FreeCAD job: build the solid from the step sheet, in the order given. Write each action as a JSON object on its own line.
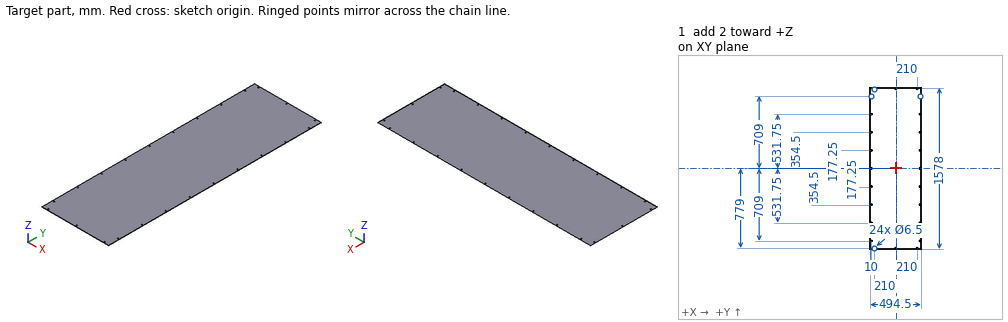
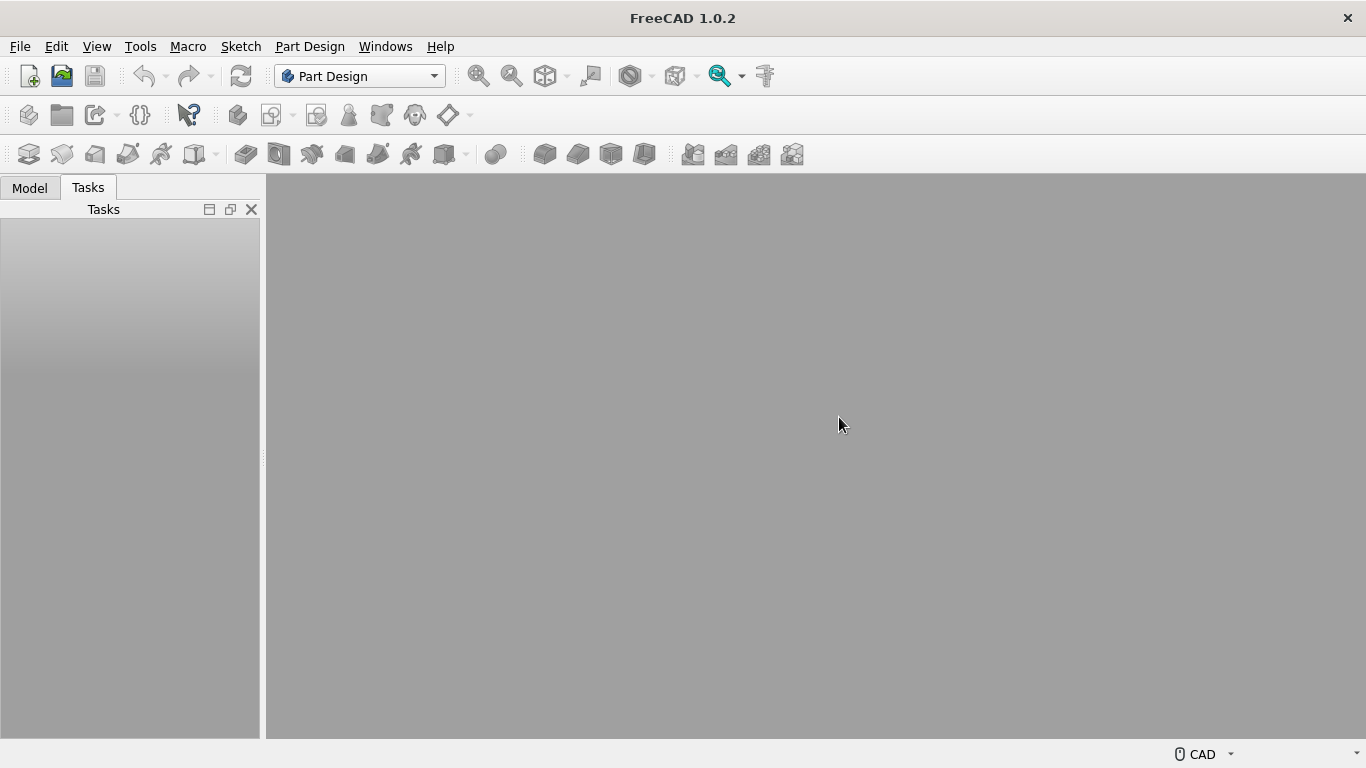
{"action": "key", "text": "ctrl+n"}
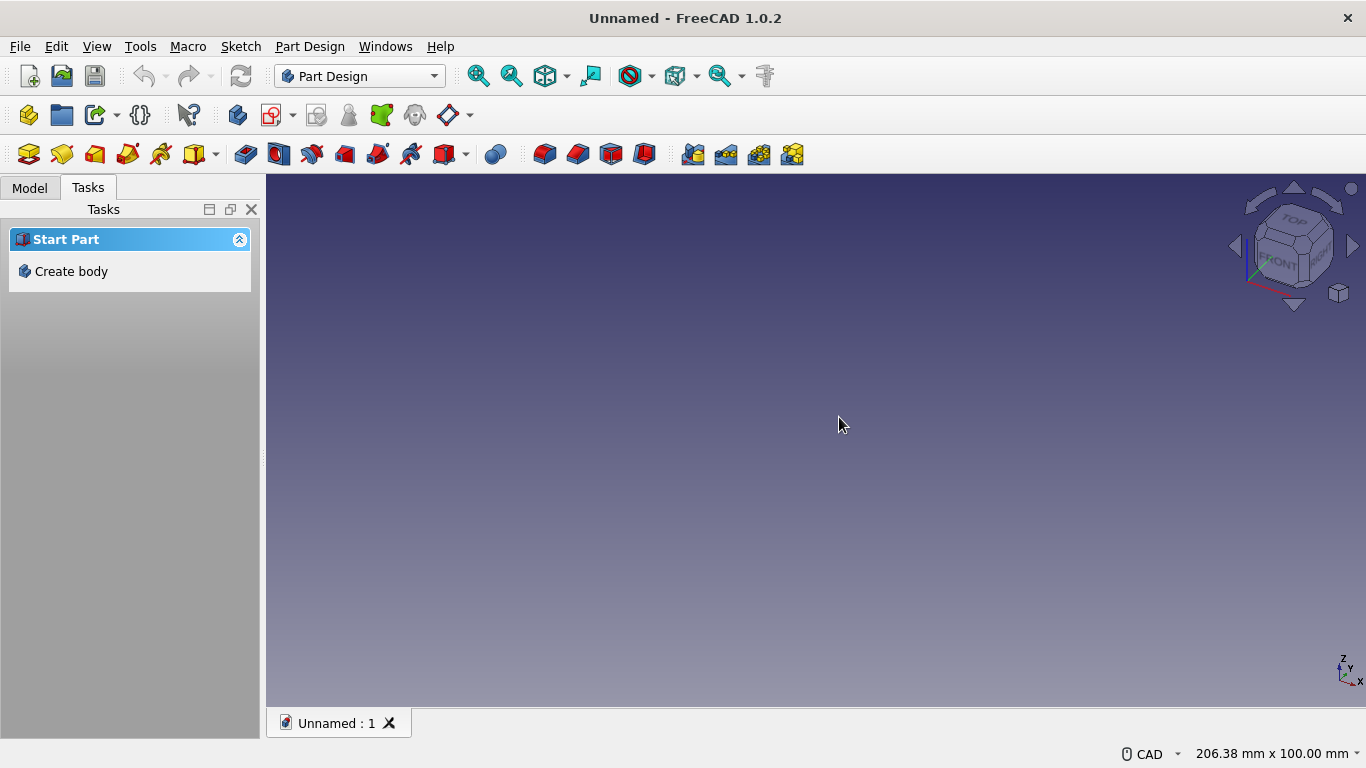
{"action": "left_click", "coordinate": [270, 116]}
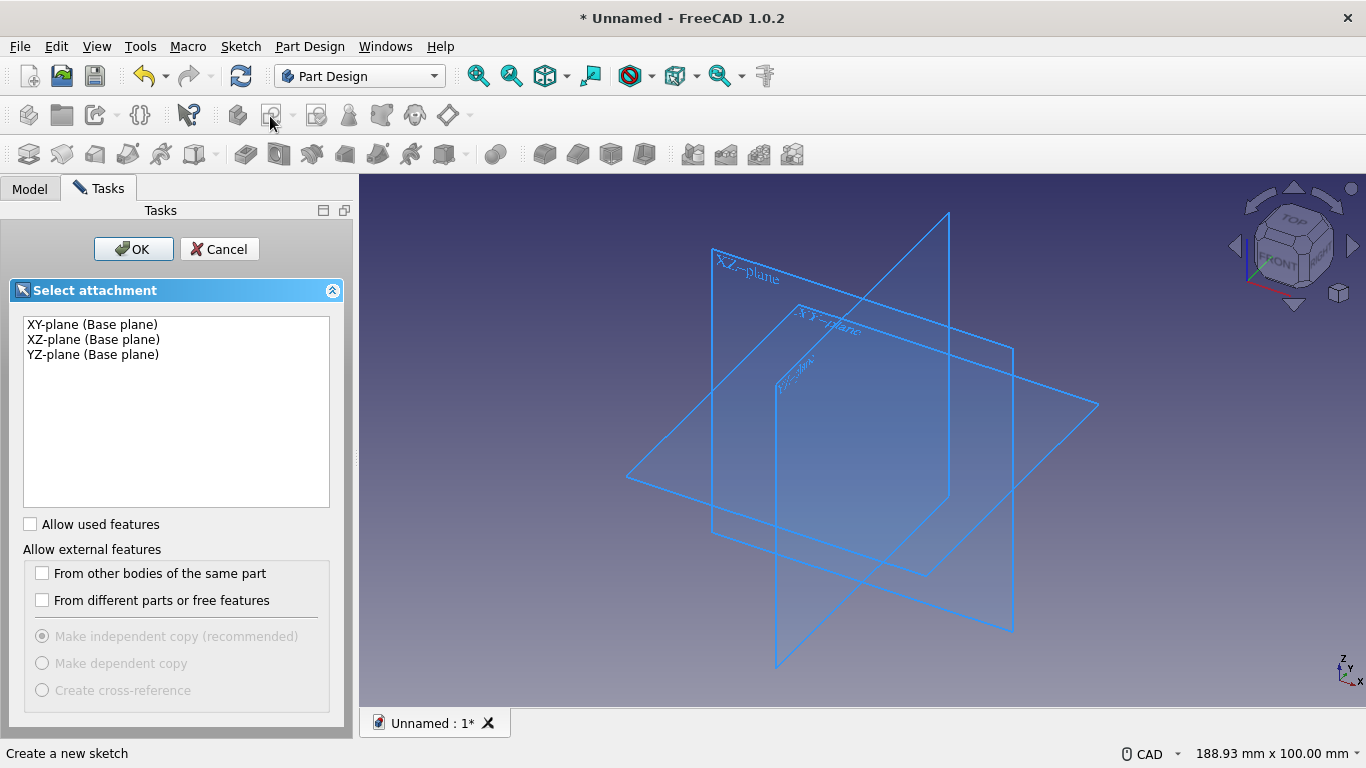
{"action": "left_click", "coordinate": [84, 324]}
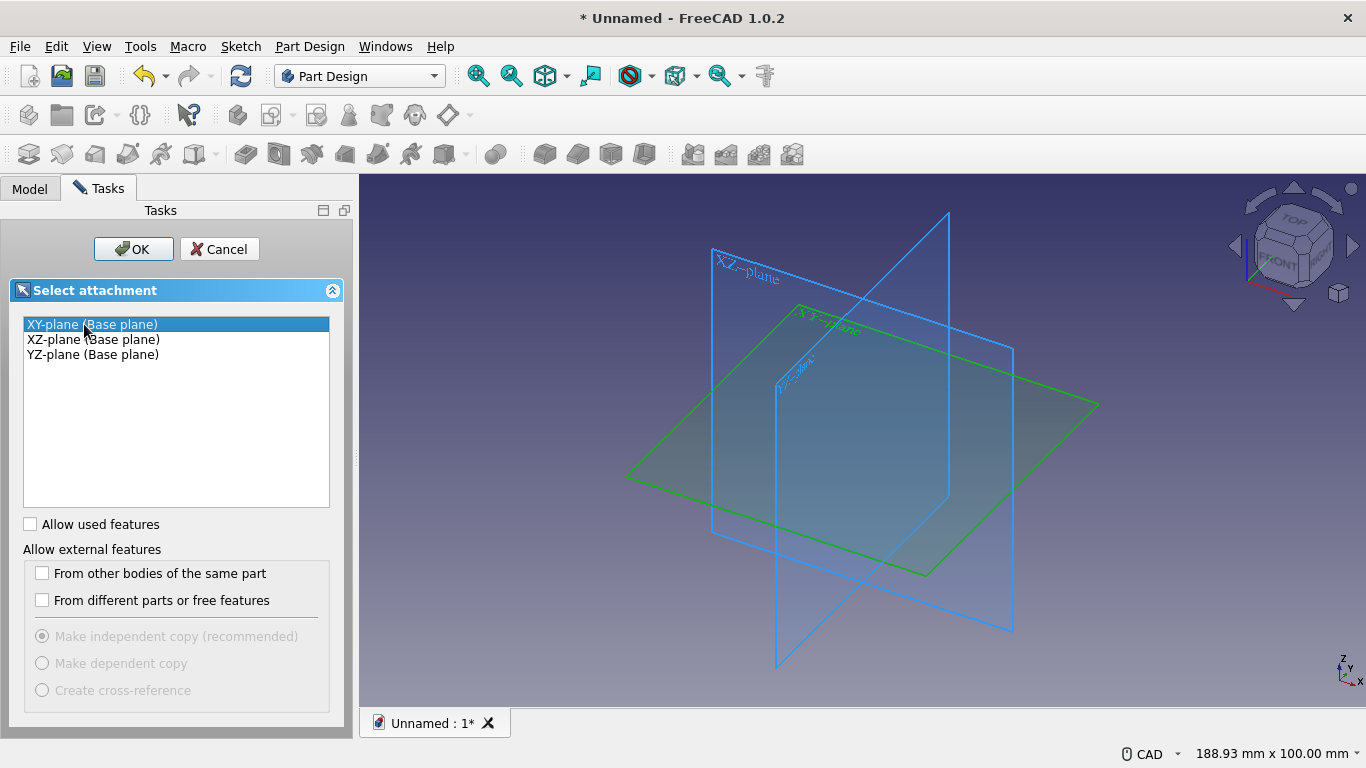
{"action": "left_click", "coordinate": [134, 249]}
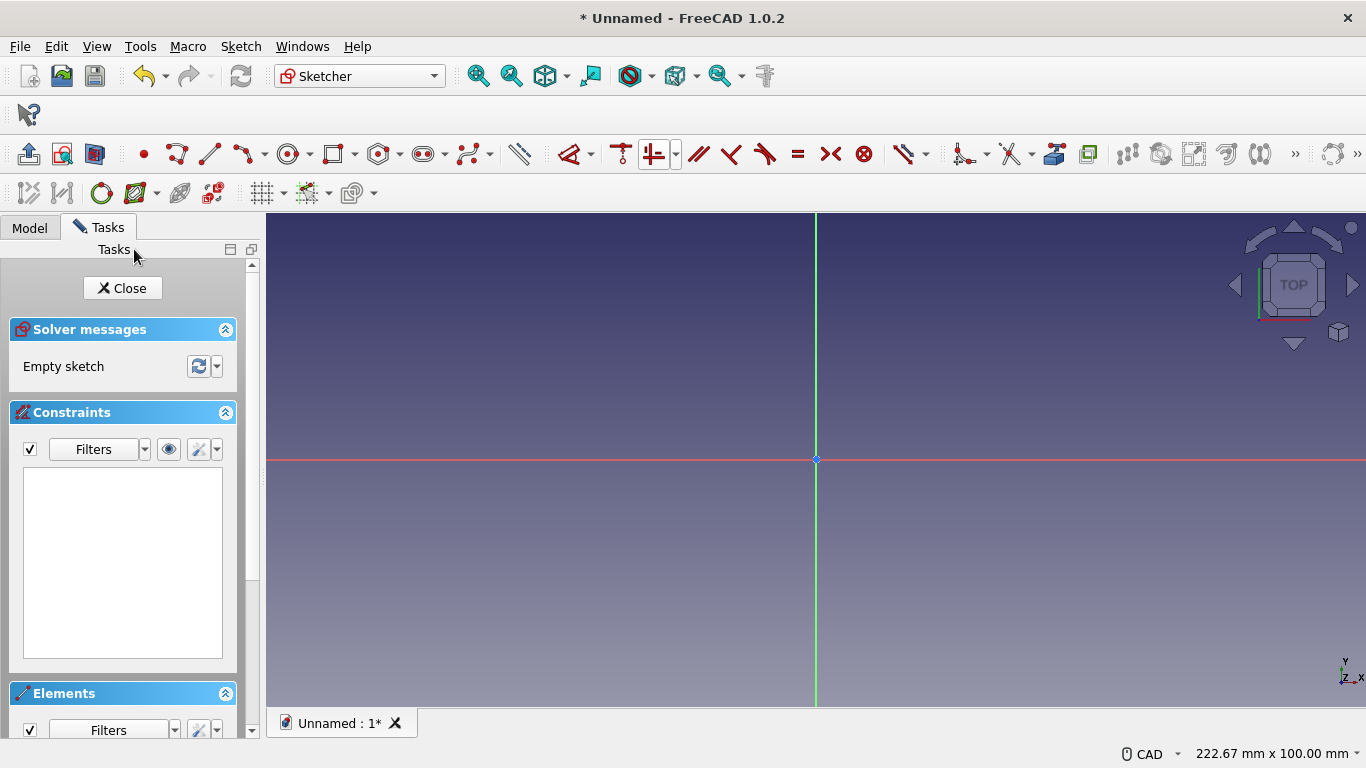
{"action": "scroll", "coordinate": [745, 460], "scroll_direction": "down", "scroll_amount": 16}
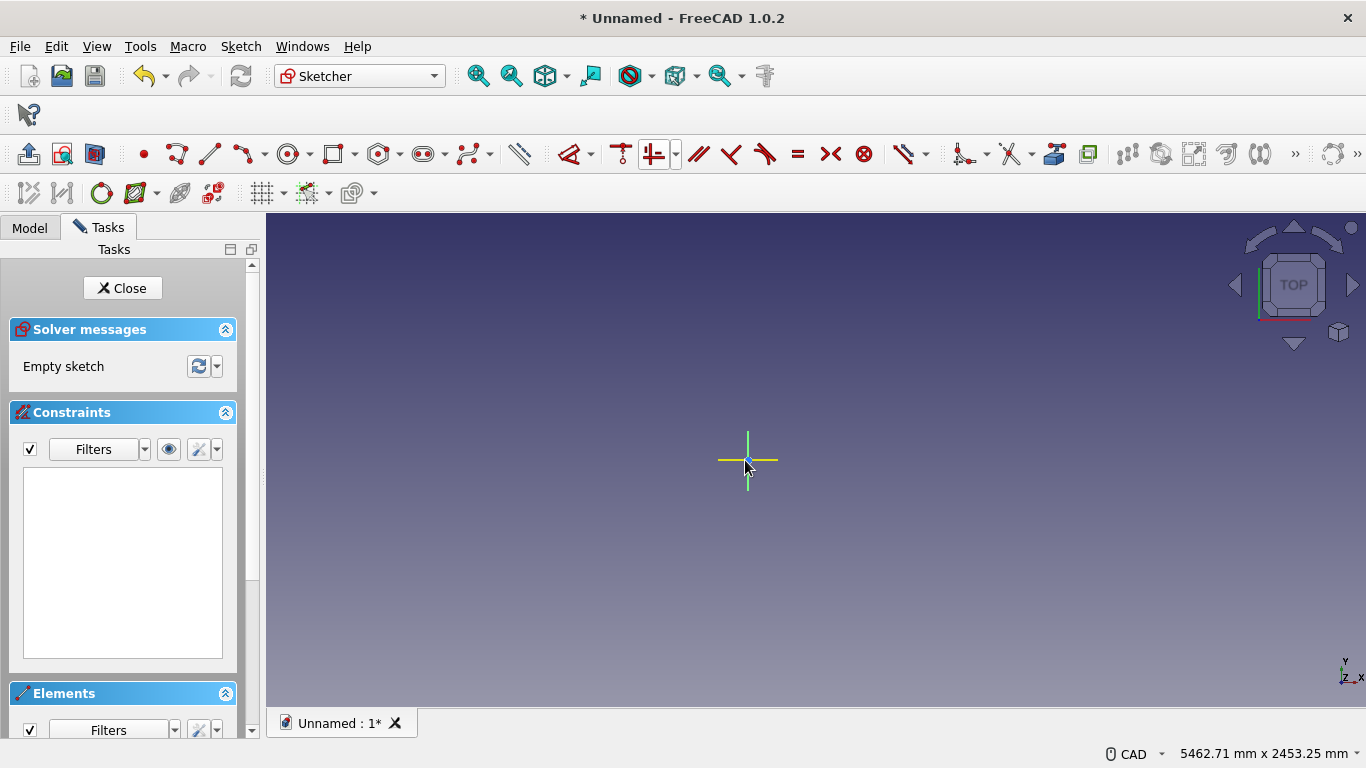
{"action": "key", "text": "g v"}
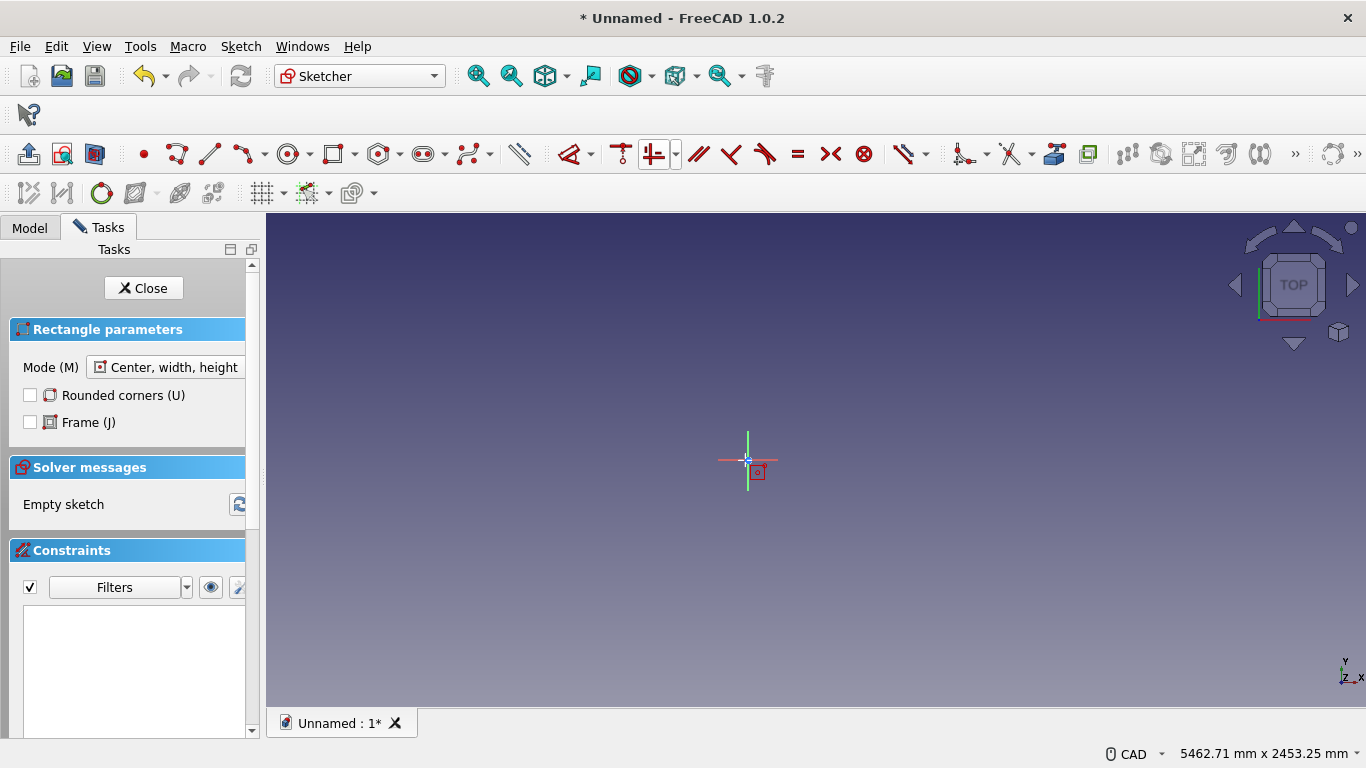
{"action": "left_click", "coordinate": [748, 460]}
{"action": "mouse_move", "coordinate": [798, 302]}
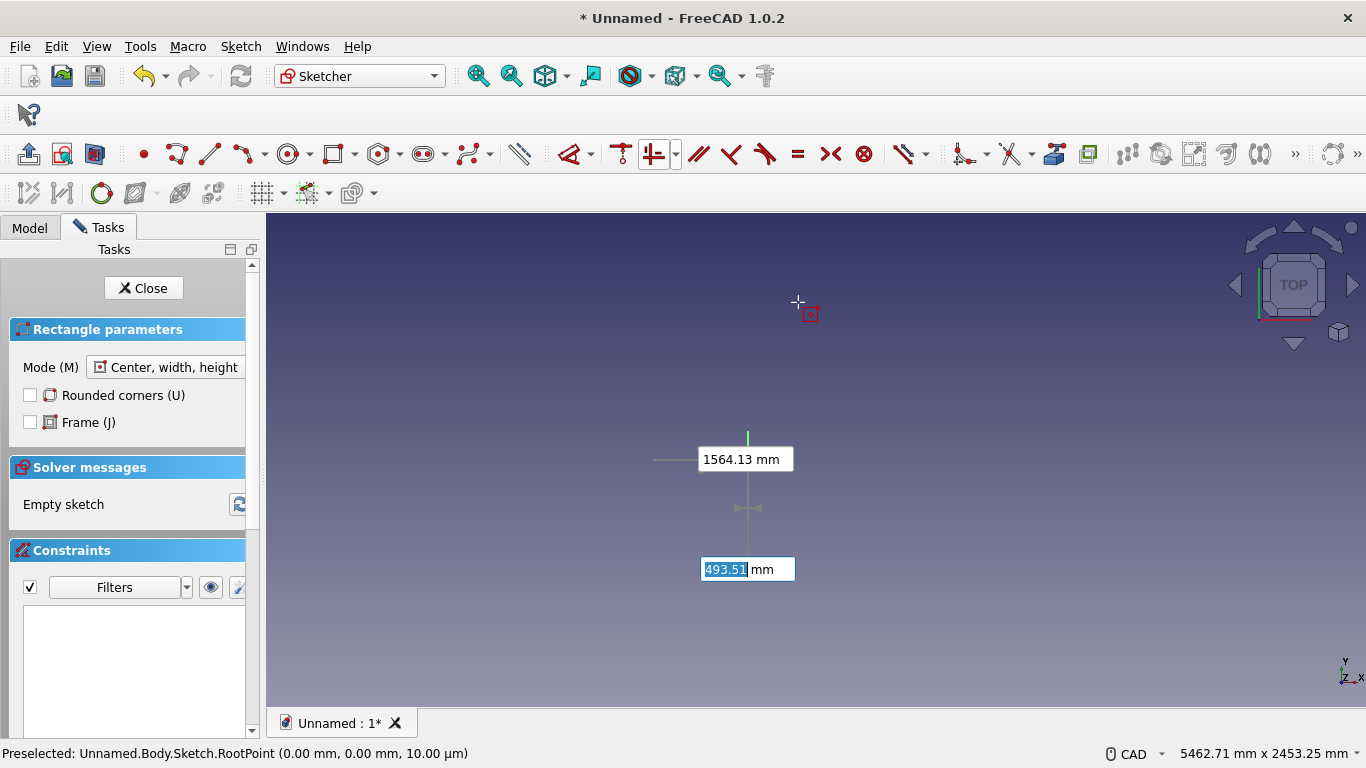
{"action": "type", "text": "494.5"}
{"action": "key", "text": "Tab"}
{"action": "type", "text": "1578"}
{"action": "key", "text": "Return"}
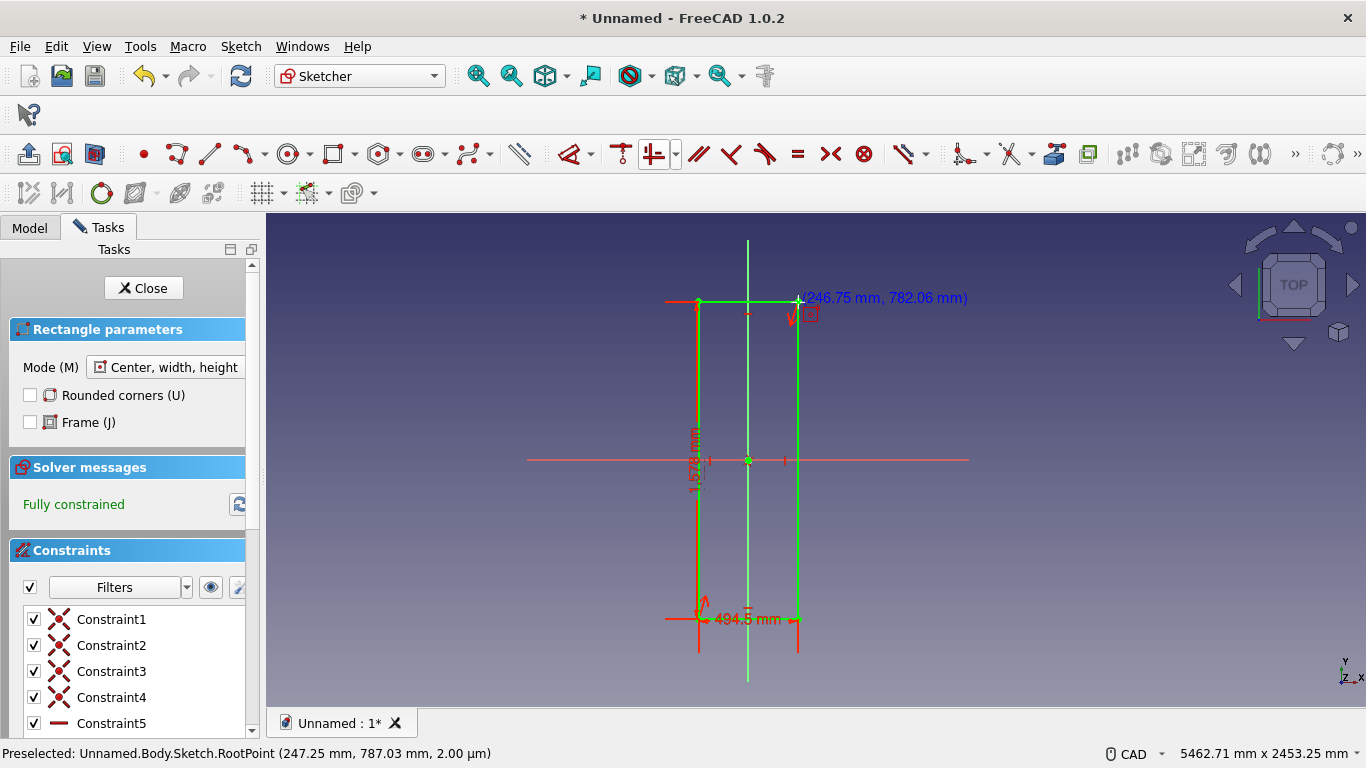
{"action": "key", "text": "g c"}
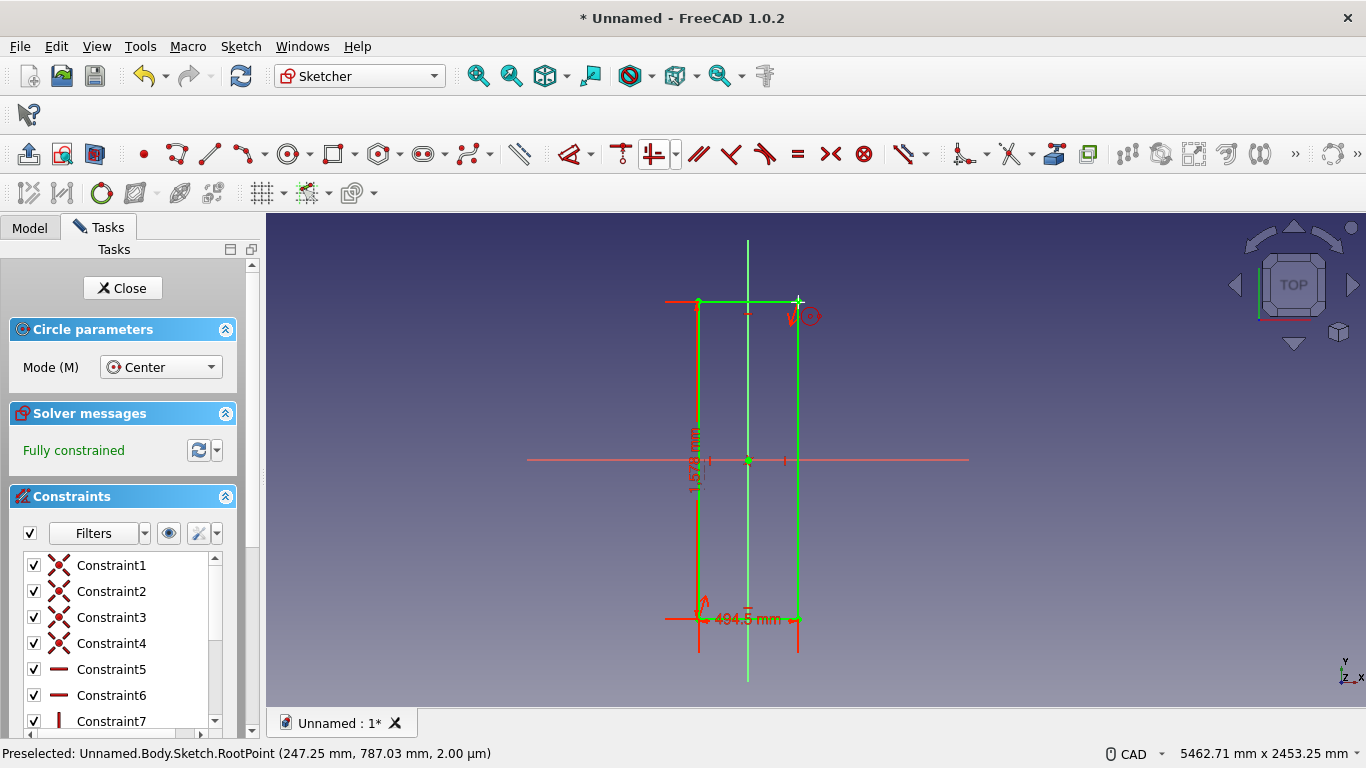
{"action": "scroll", "coordinate": [701, 603], "scroll_direction": "up", "scroll_amount": 18}